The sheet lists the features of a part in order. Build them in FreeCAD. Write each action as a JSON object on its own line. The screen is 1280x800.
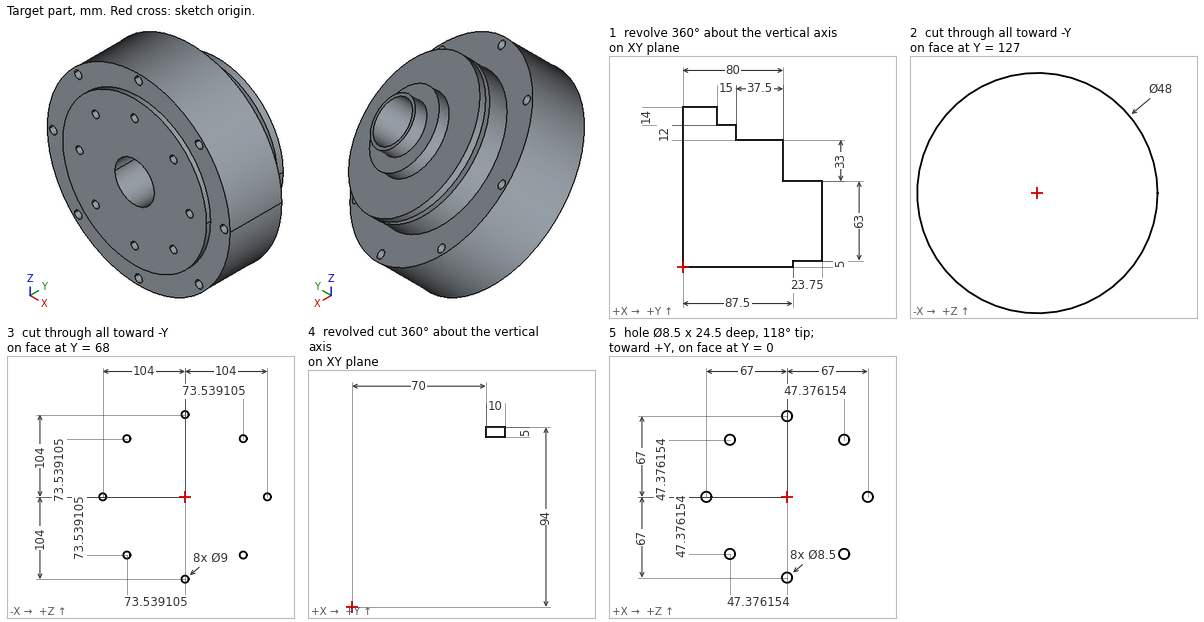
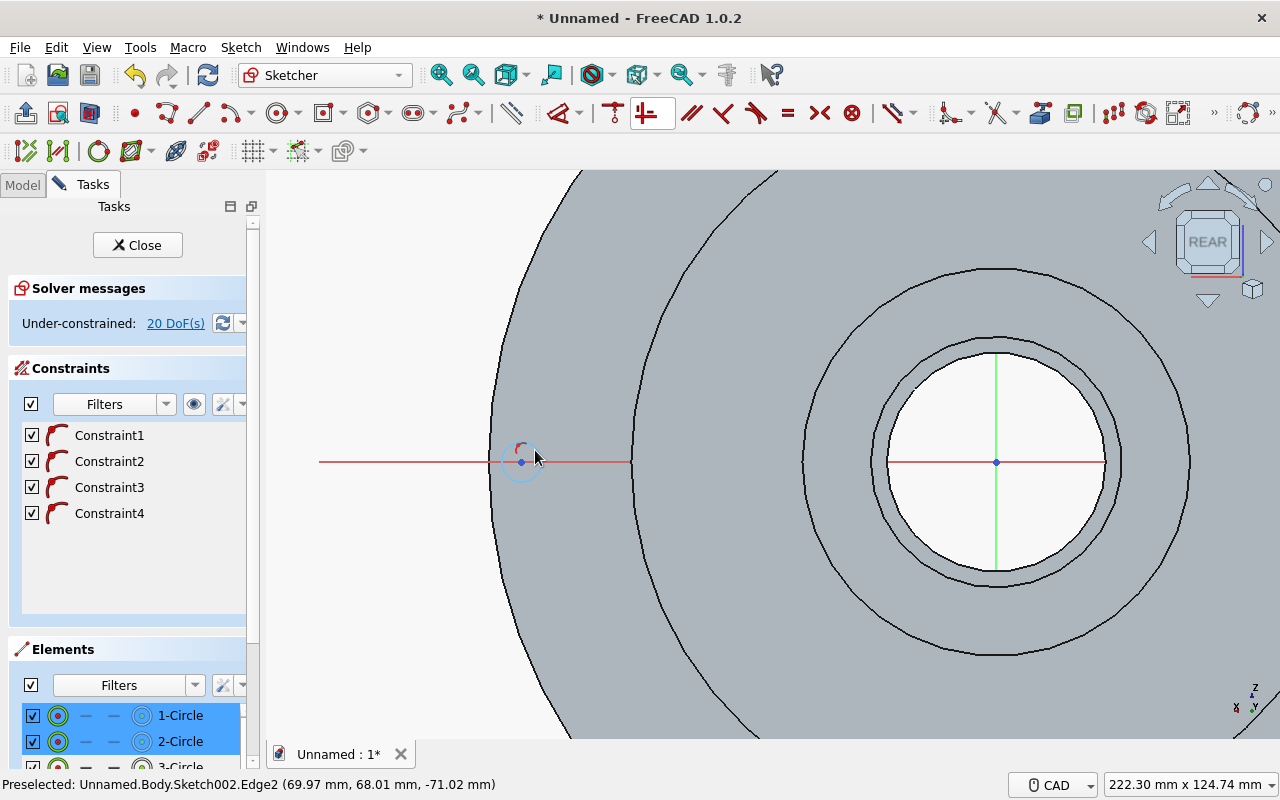
{"action": "left_click", "coordinate": [536, 448]}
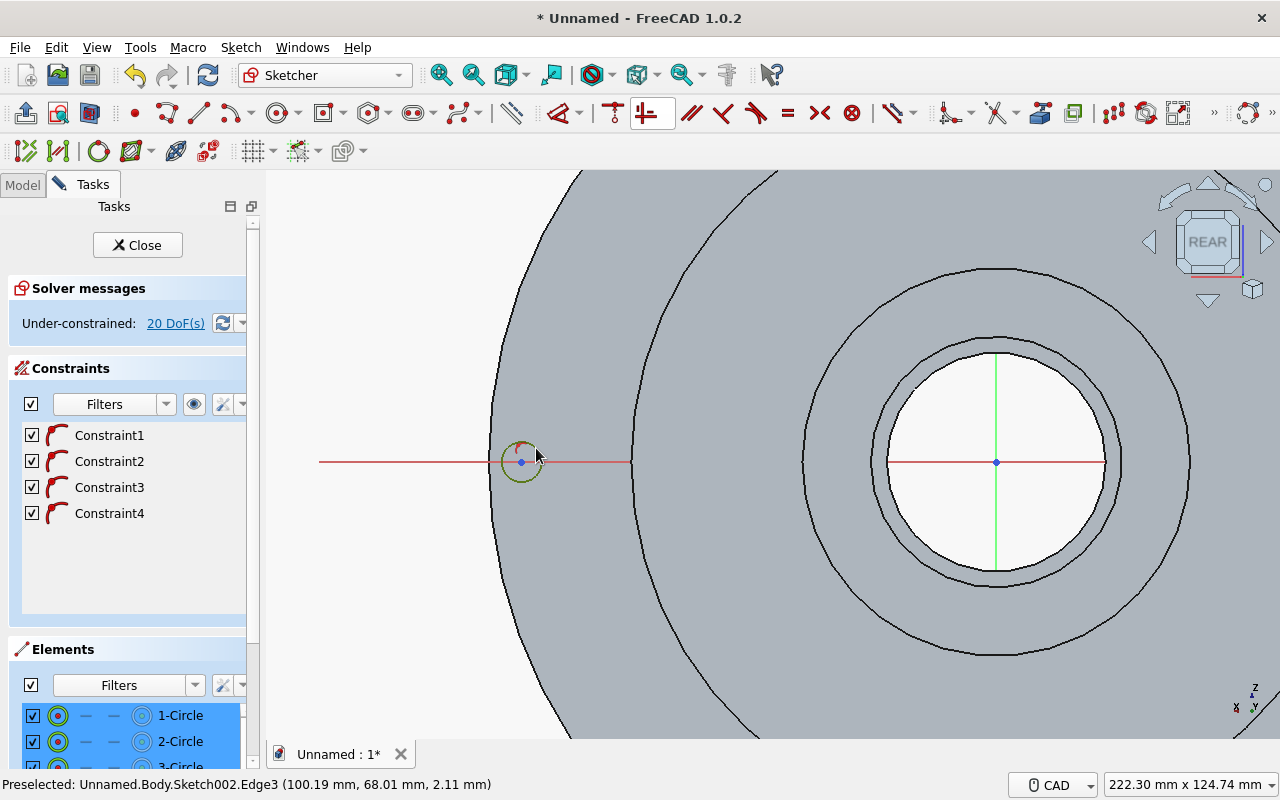
{"action": "scroll", "coordinate": [535, 450], "scroll_direction": "down", "scroll_amount": 5}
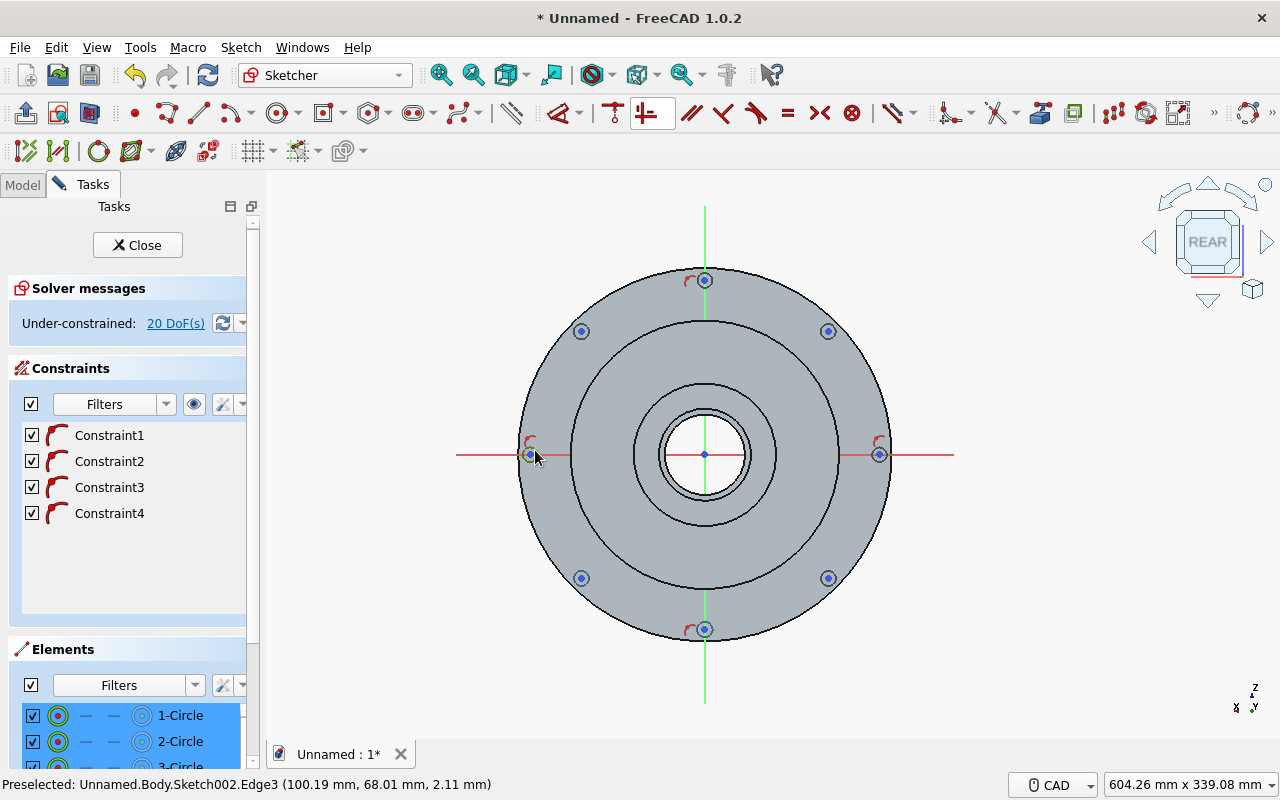
{"action": "scroll", "coordinate": [587, 326], "scroll_direction": "up", "scroll_amount": 3}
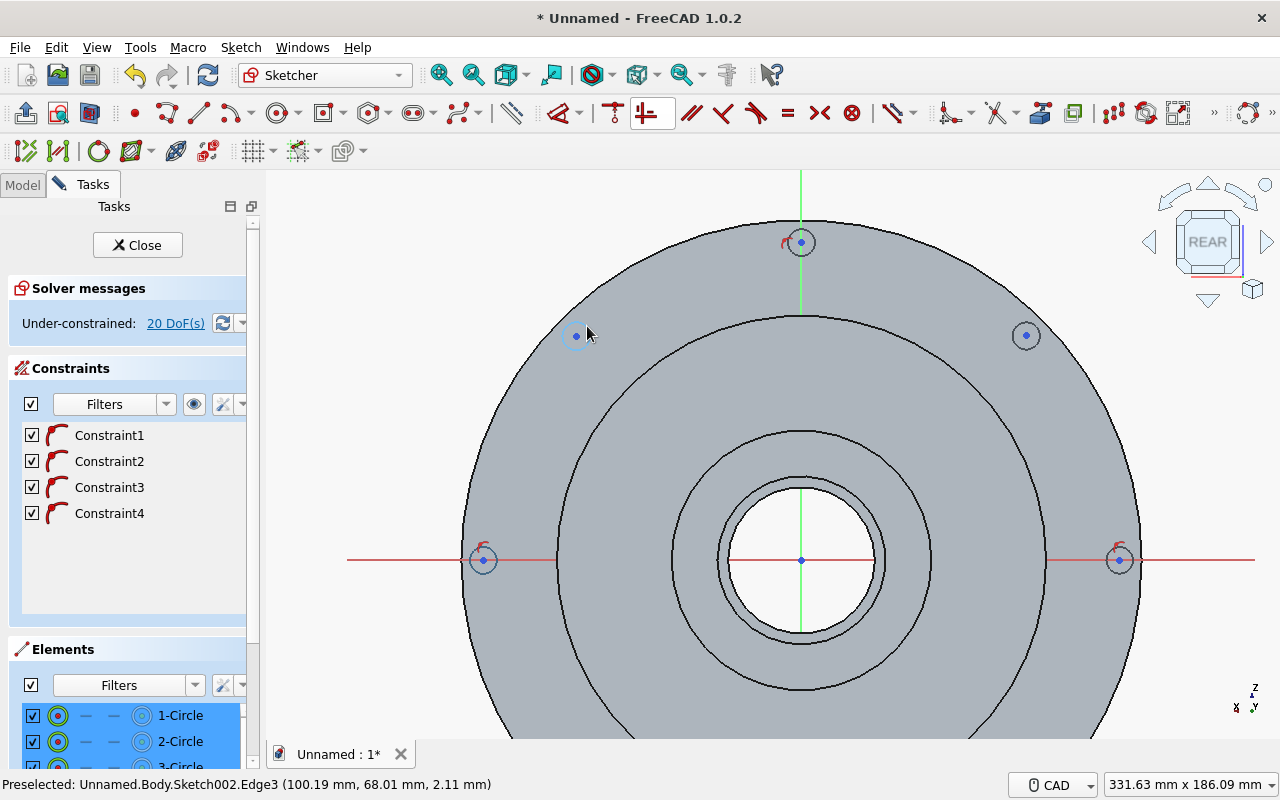
{"action": "left_click", "coordinate": [586, 326]}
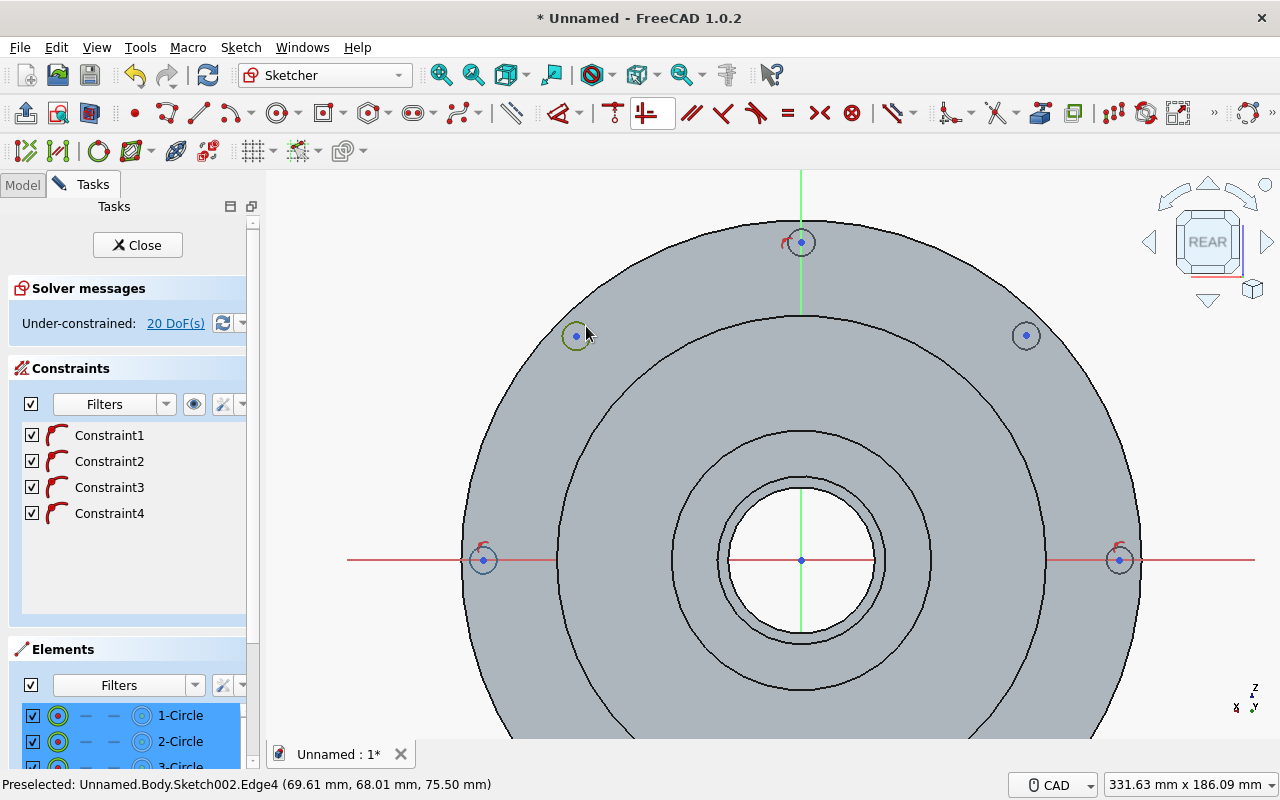
{"action": "scroll", "coordinate": [811, 233], "scroll_direction": "up", "scroll_amount": 2}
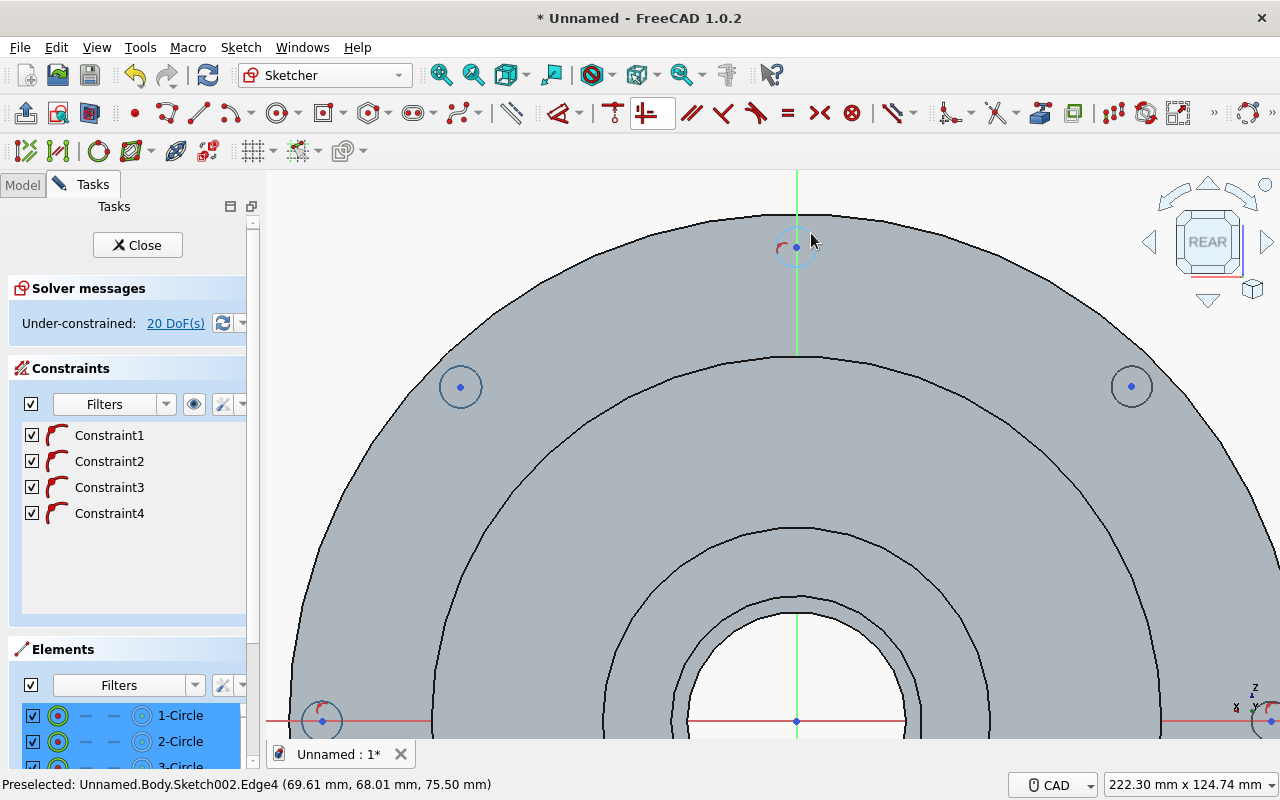
{"action": "left_click", "coordinate": [811, 233]}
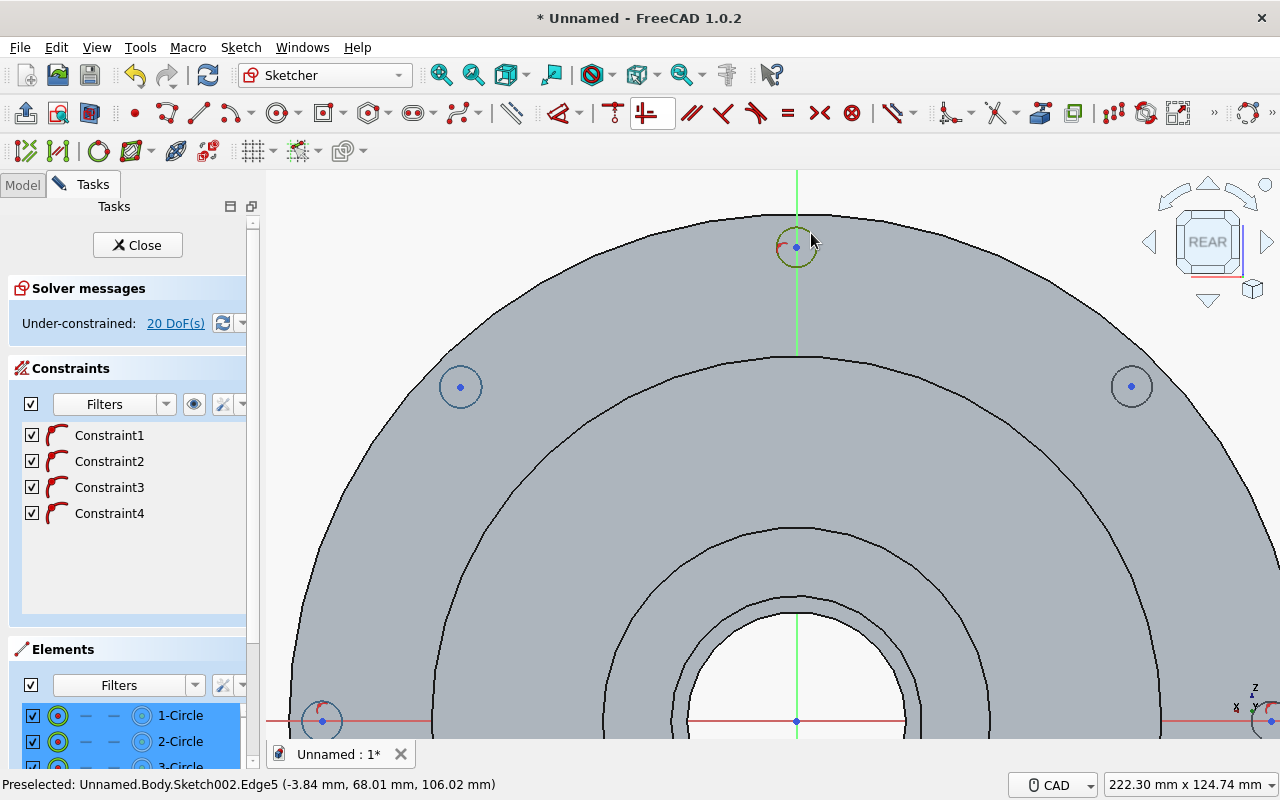
{"action": "left_click", "coordinate": [1112, 386]}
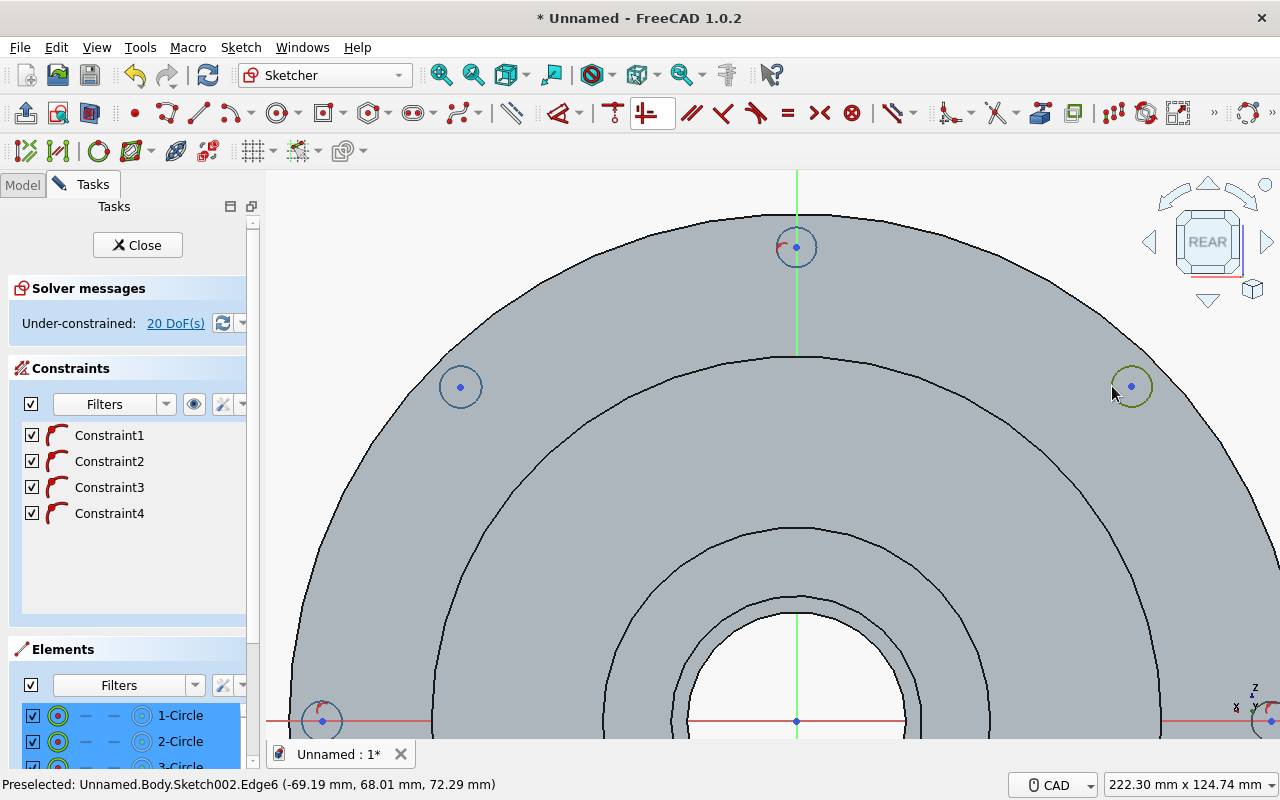
{"action": "scroll", "coordinate": [651, 299], "scroll_direction": "down", "scroll_amount": 5}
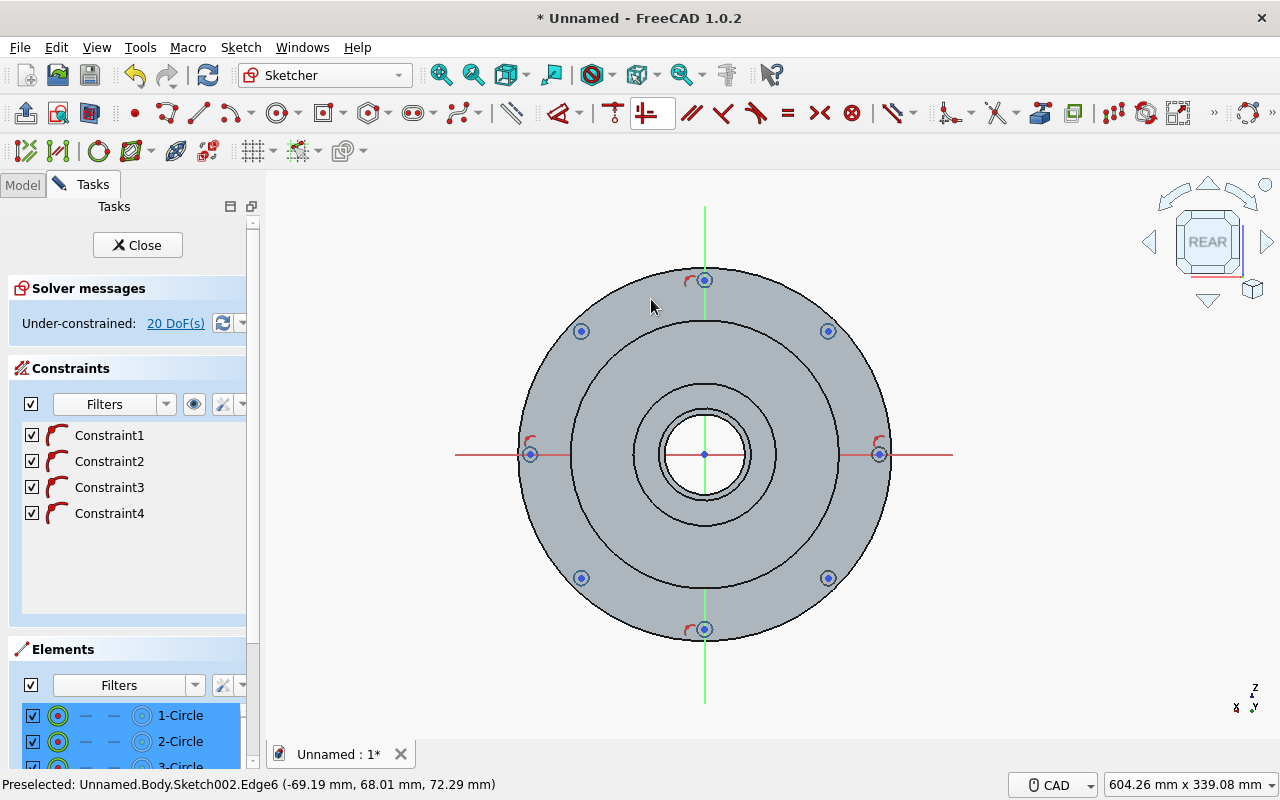
{"action": "scroll", "coordinate": [885, 449], "scroll_direction": "up", "scroll_amount": 5}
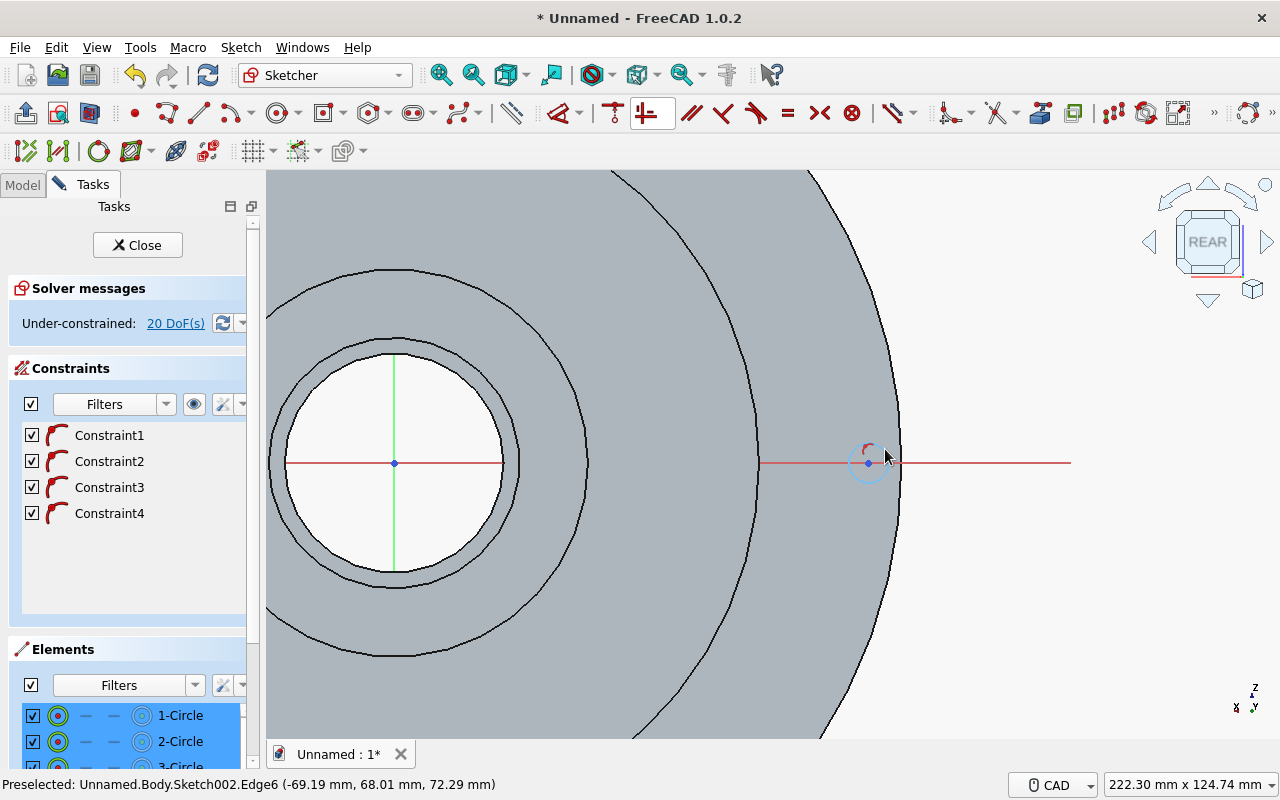
{"action": "left_click", "coordinate": [883, 449]}